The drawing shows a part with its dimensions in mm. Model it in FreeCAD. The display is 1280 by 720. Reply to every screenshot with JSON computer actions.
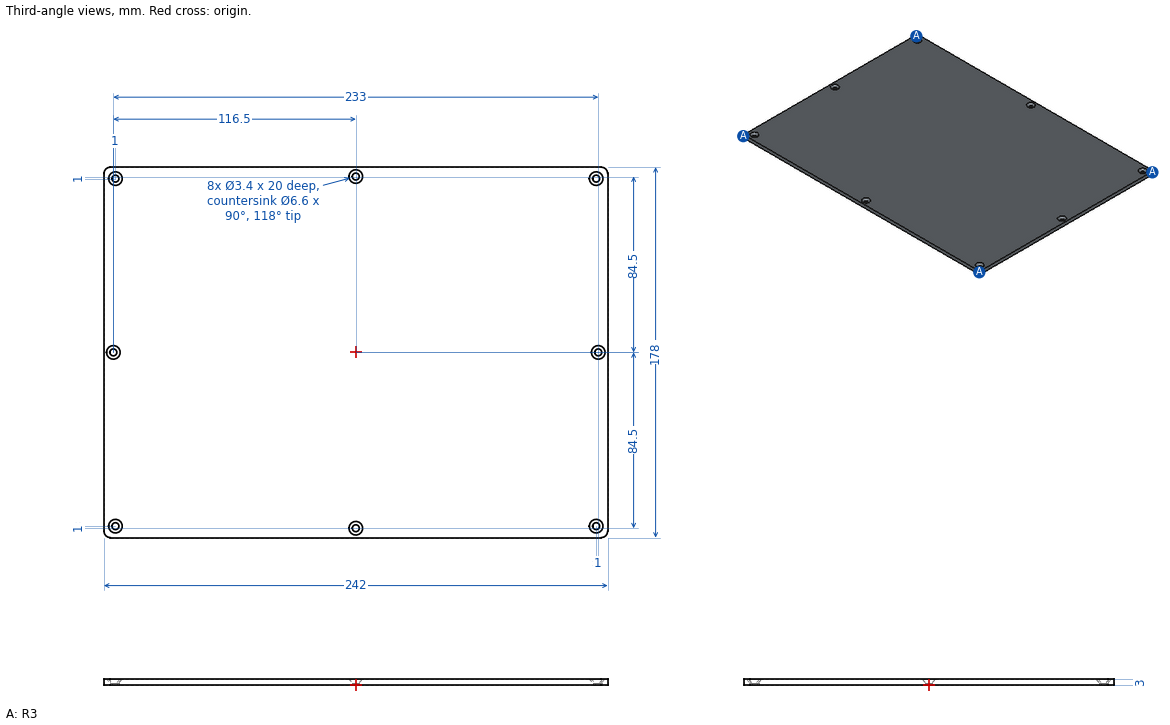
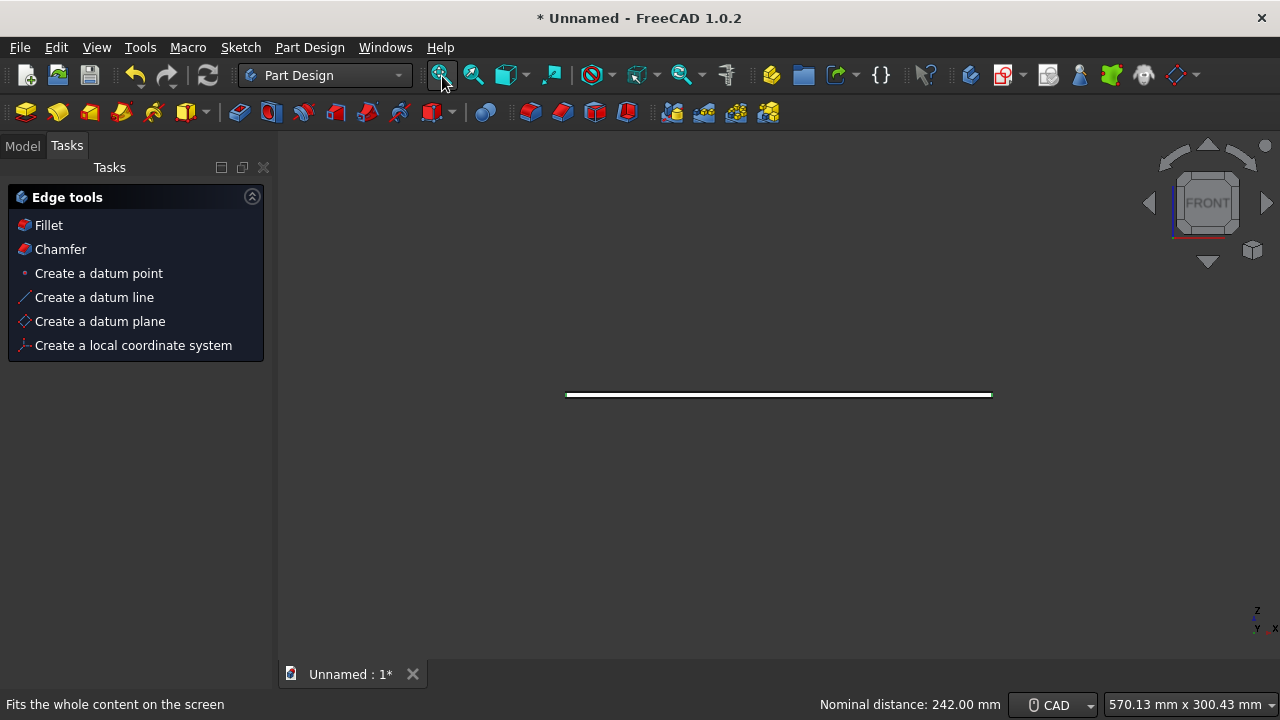
{"action": "key", "text": "3"}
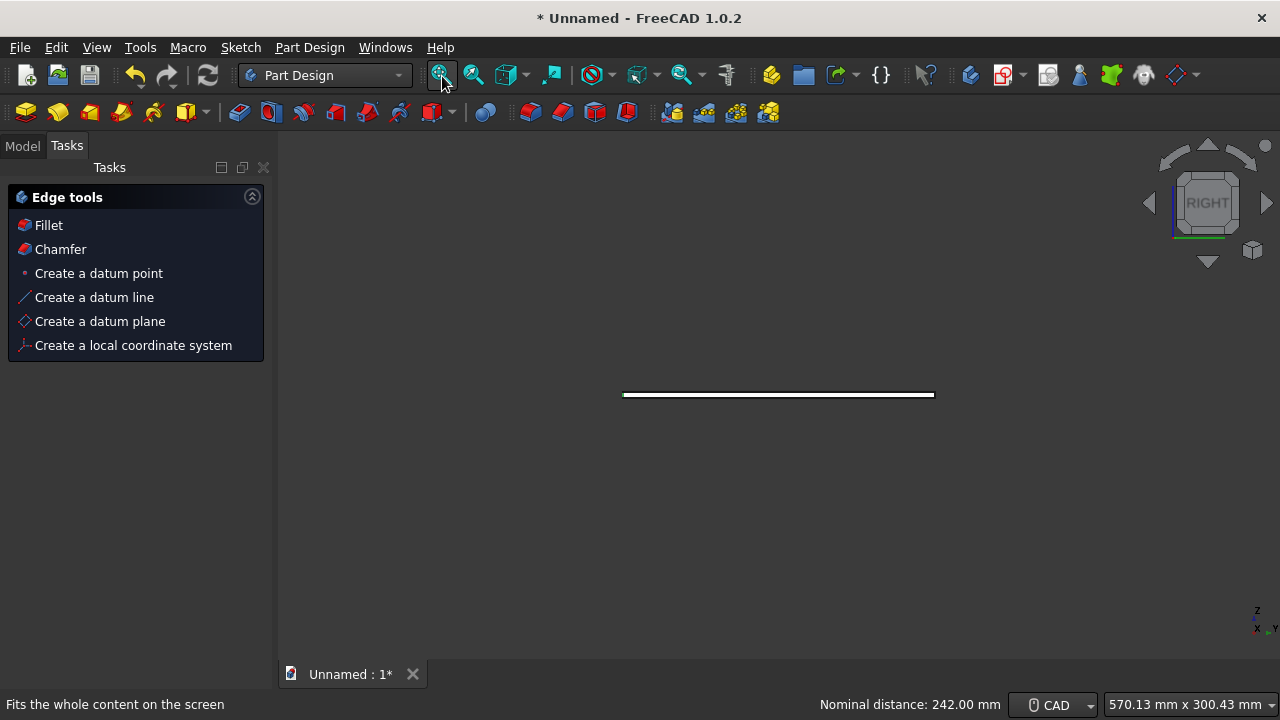
{"action": "left_click", "coordinate": [442, 76]}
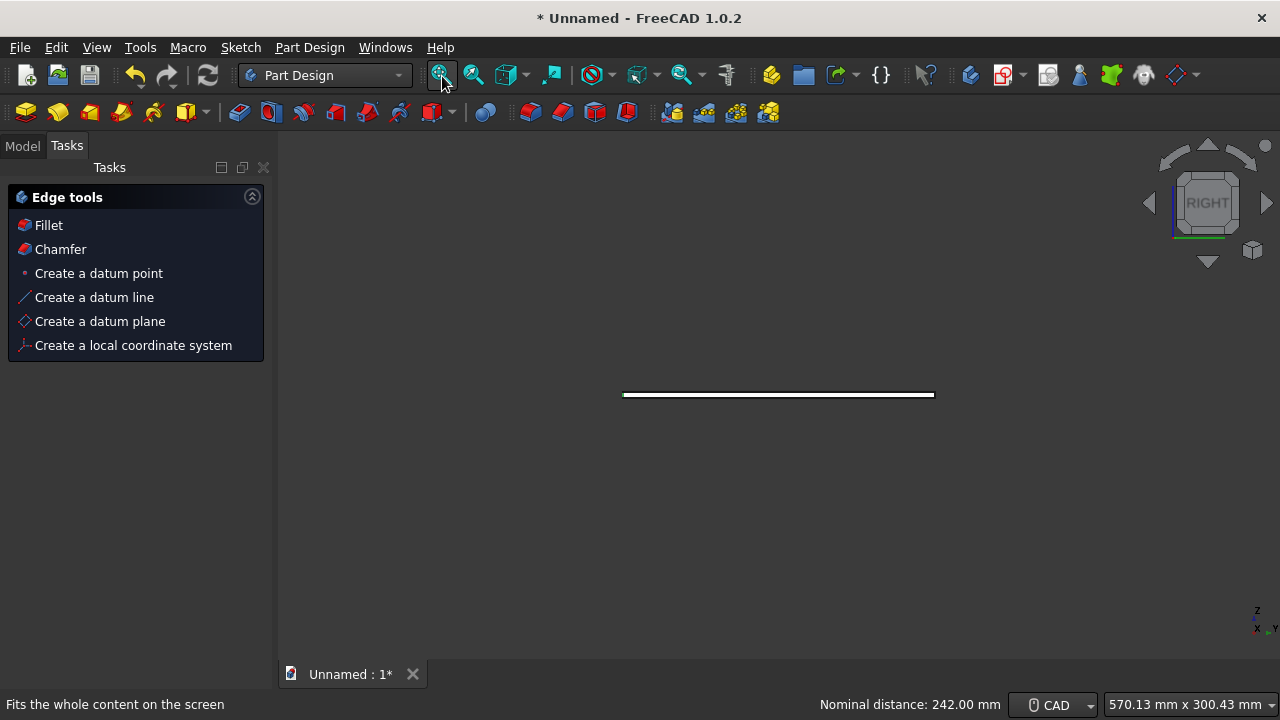
{"action": "scroll", "coordinate": [935, 394], "scroll_direction": "up", "scroll_amount": 11}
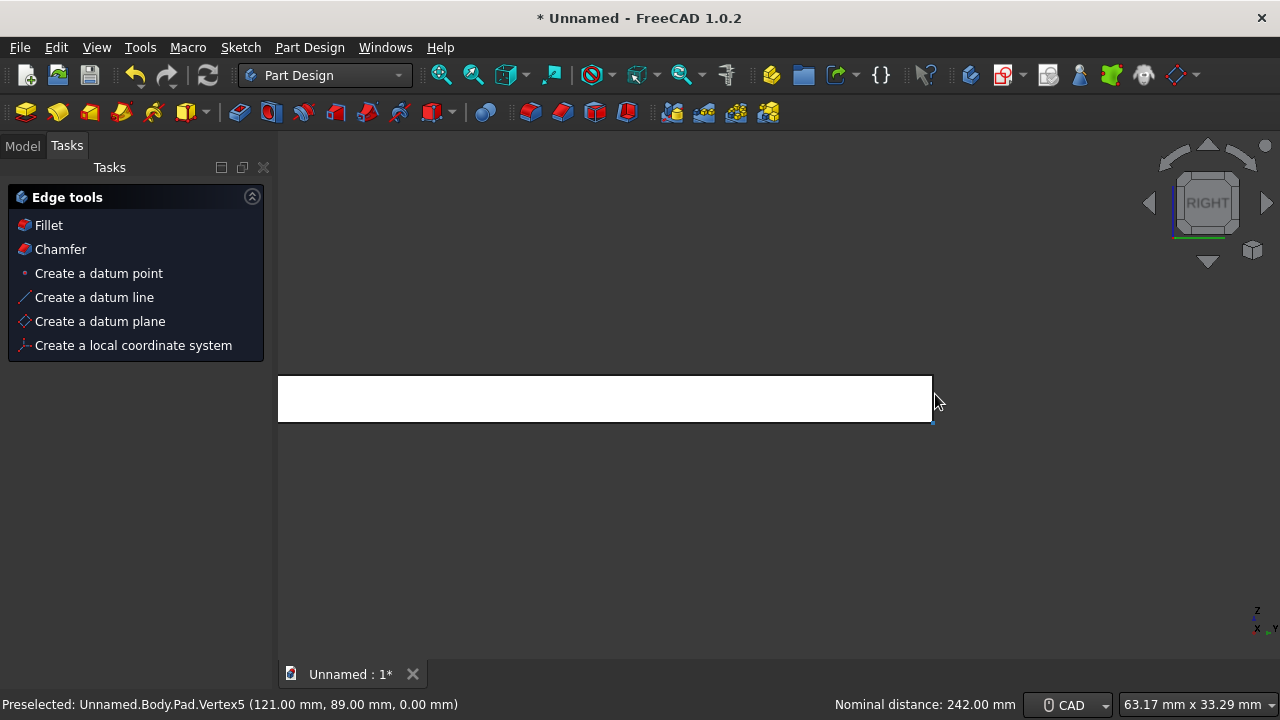
{"action": "left_click", "coordinate": [933, 398], "text": "ctrl"}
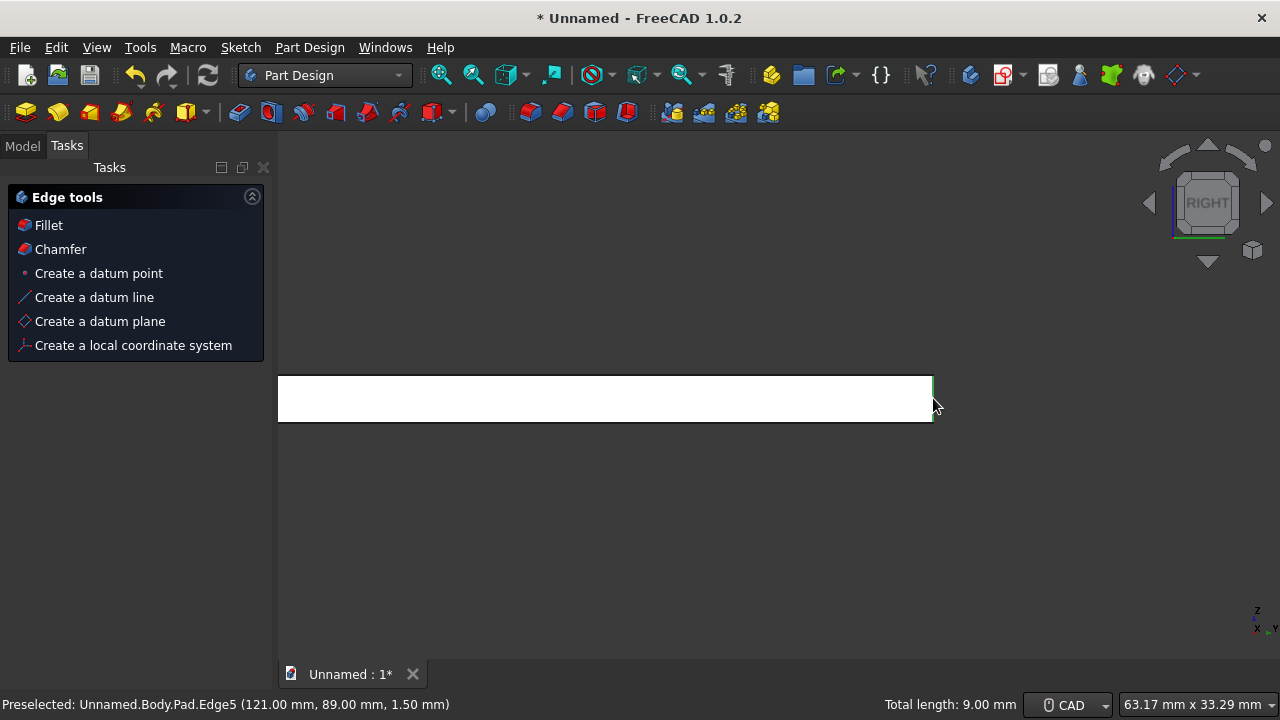
{"action": "left_click", "coordinate": [442, 76]}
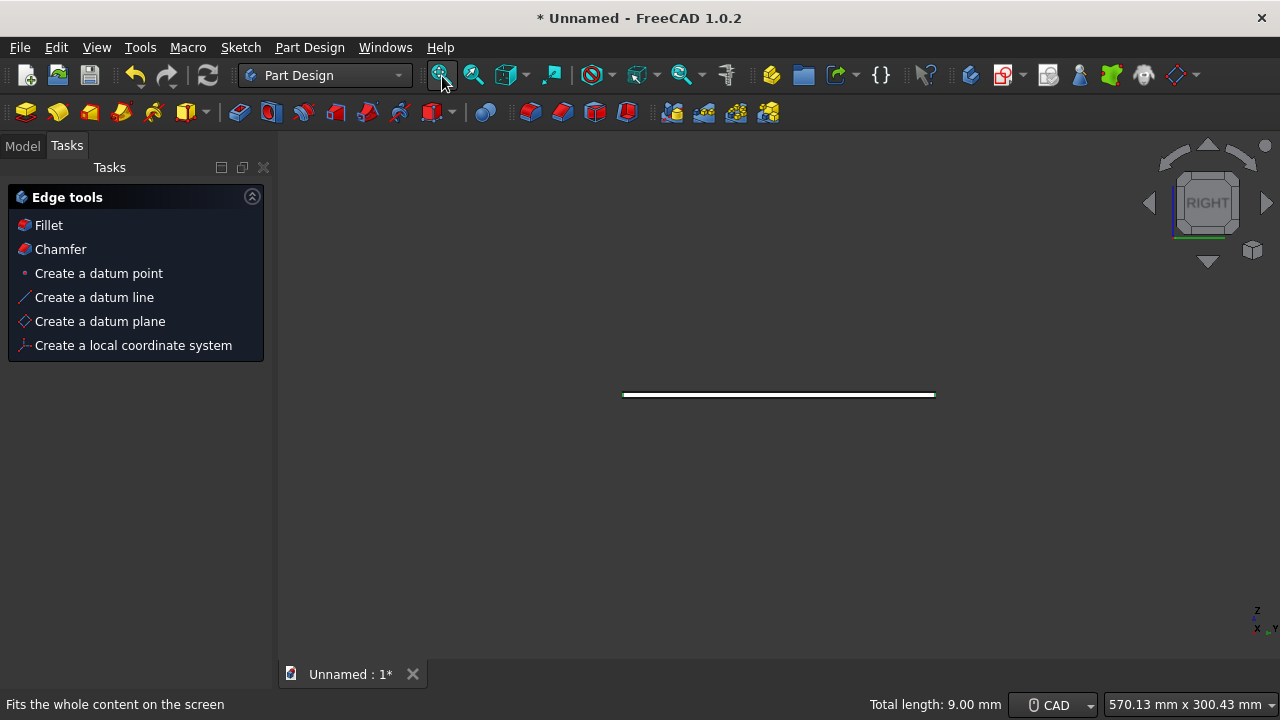
{"action": "key", "text": "5"}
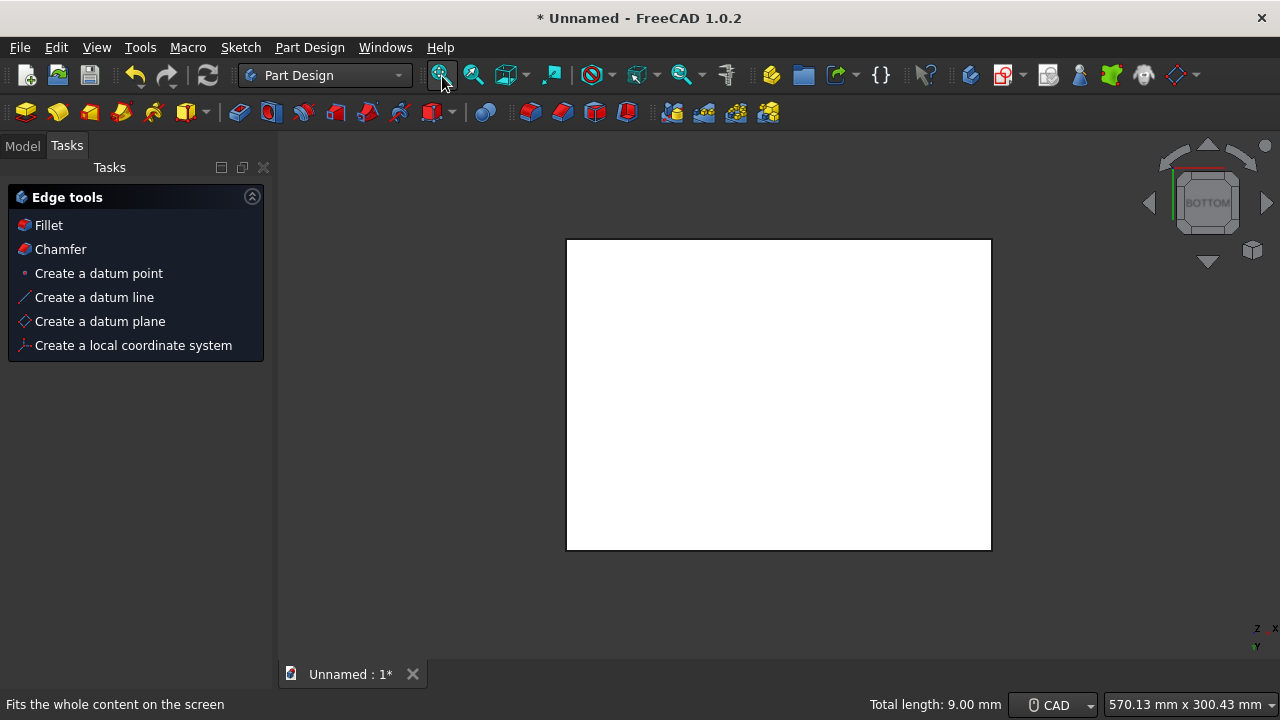
{"action": "scroll", "coordinate": [566, 550], "scroll_direction": "up", "scroll_amount": 11}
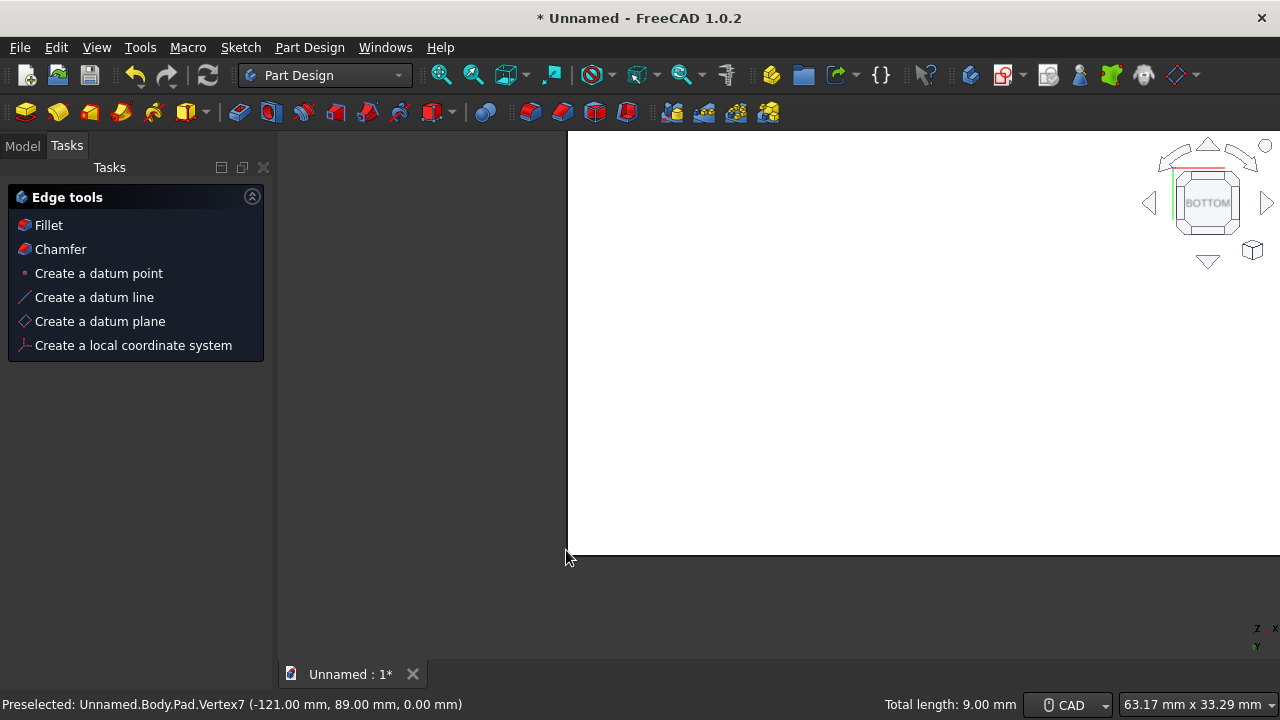
{"action": "left_click", "coordinate": [442, 76]}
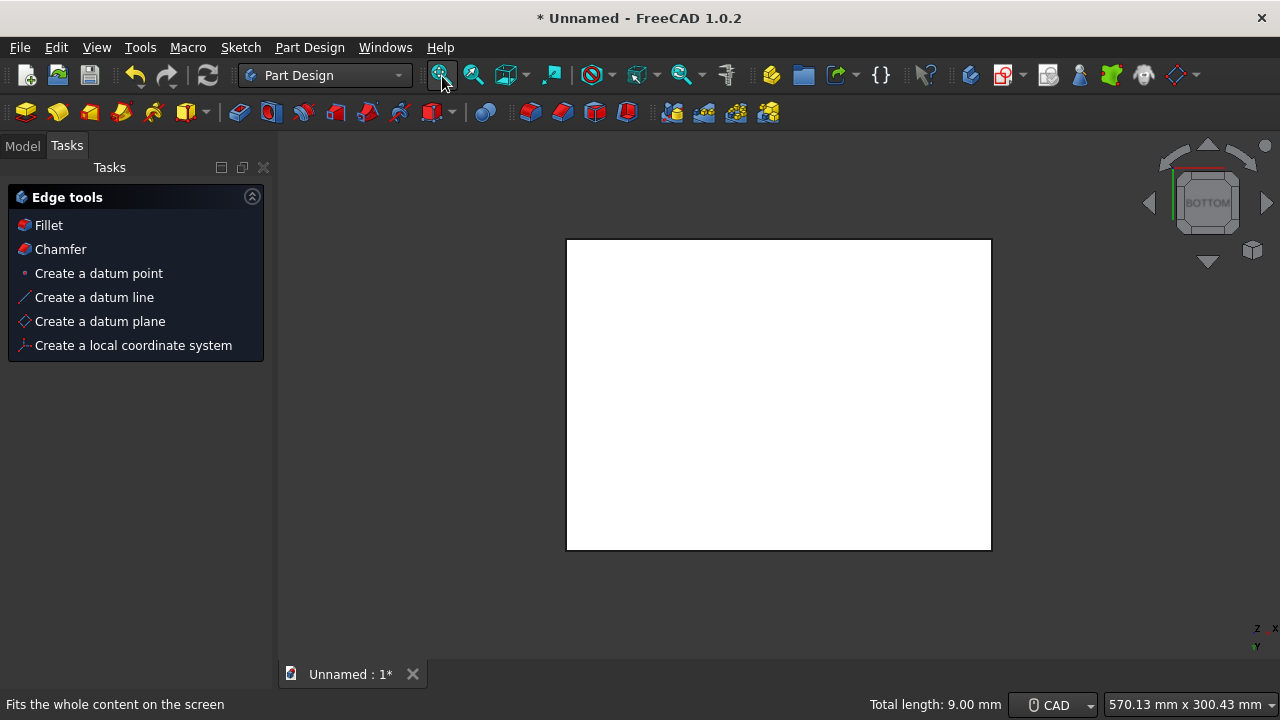
{"action": "key", "text": "4"}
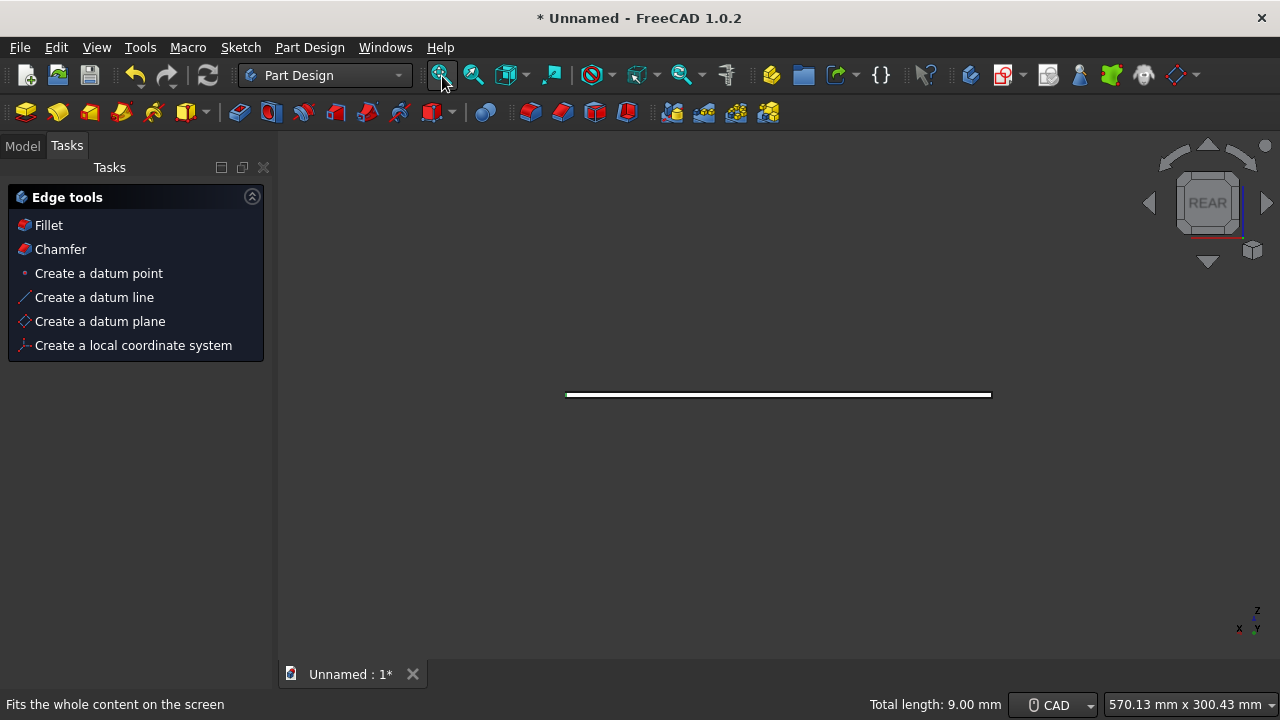
{"action": "key", "text": "v f"}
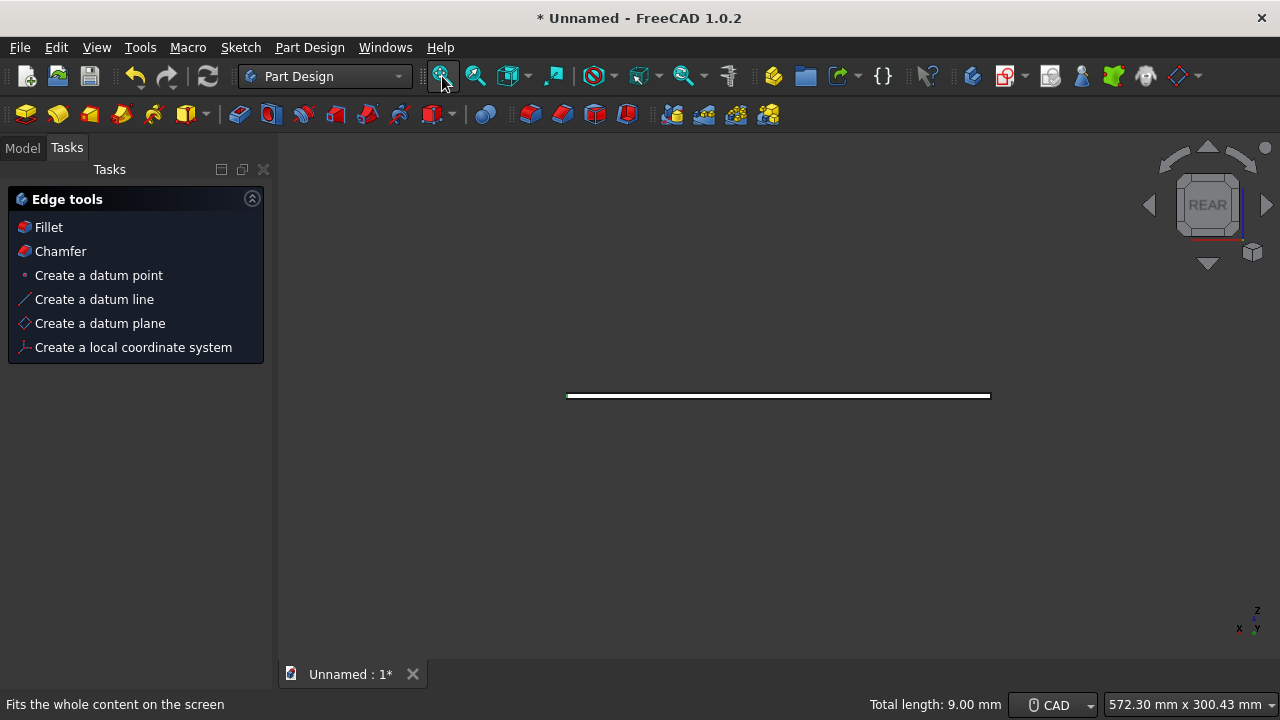
{"action": "scroll", "coordinate": [991, 395], "scroll_direction": "up", "scroll_amount": 11}